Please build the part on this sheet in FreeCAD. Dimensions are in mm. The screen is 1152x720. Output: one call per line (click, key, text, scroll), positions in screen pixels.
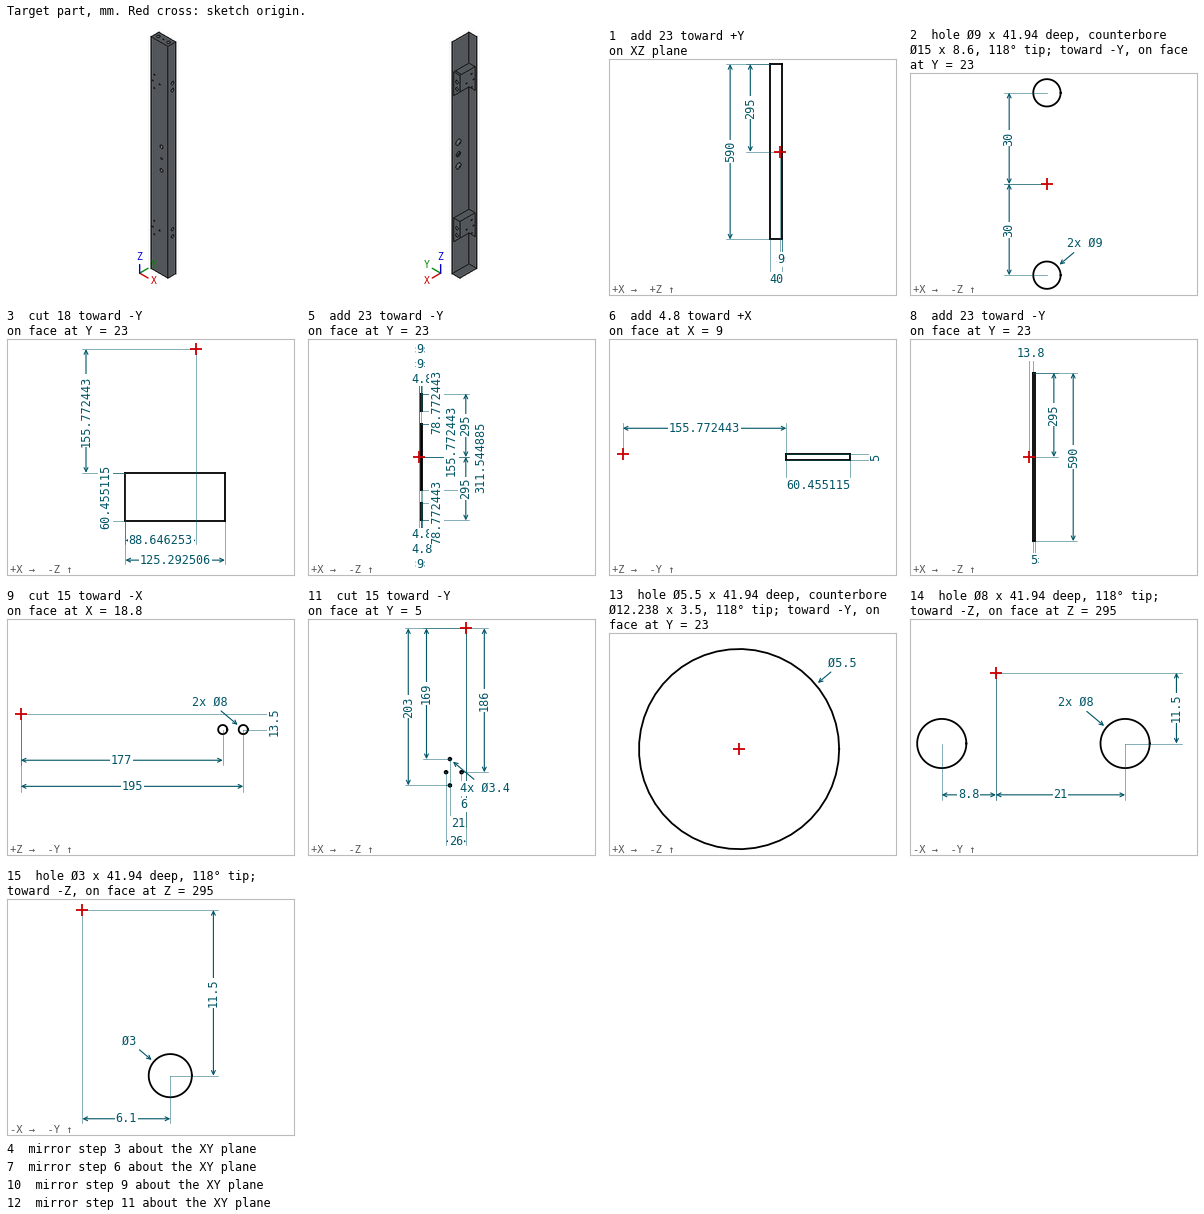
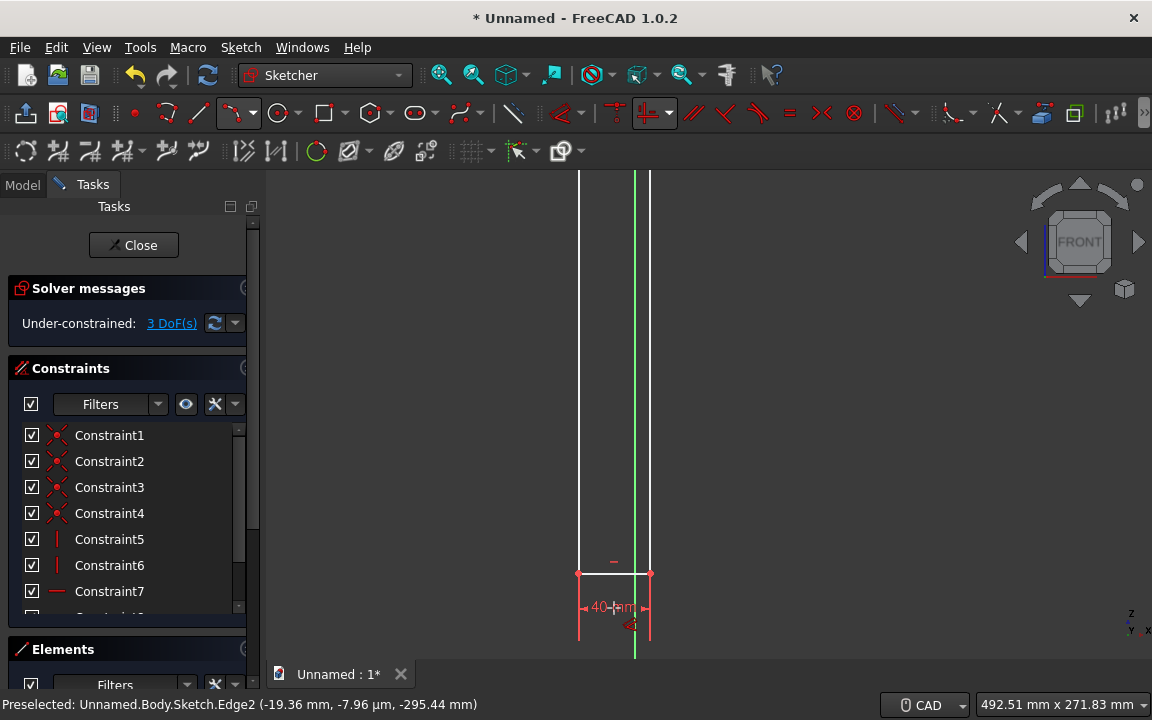
scroll(650, 574, up, 5)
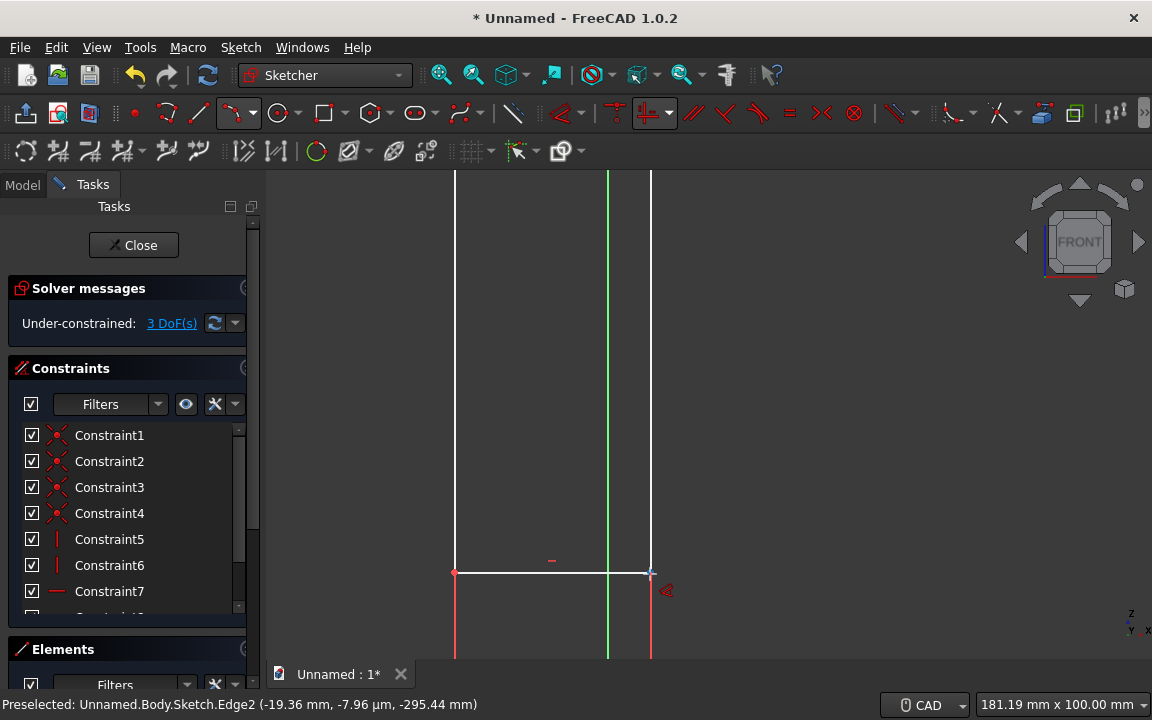
click(651, 573)
click(629, 607)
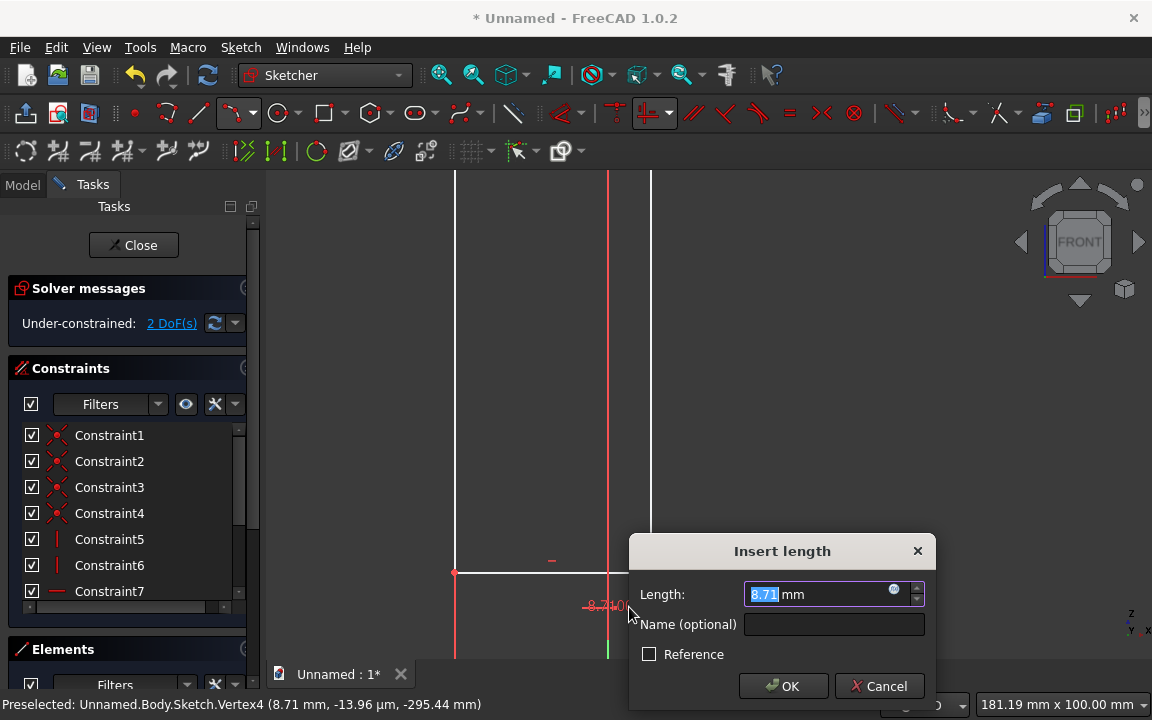
text(9)
key(Return)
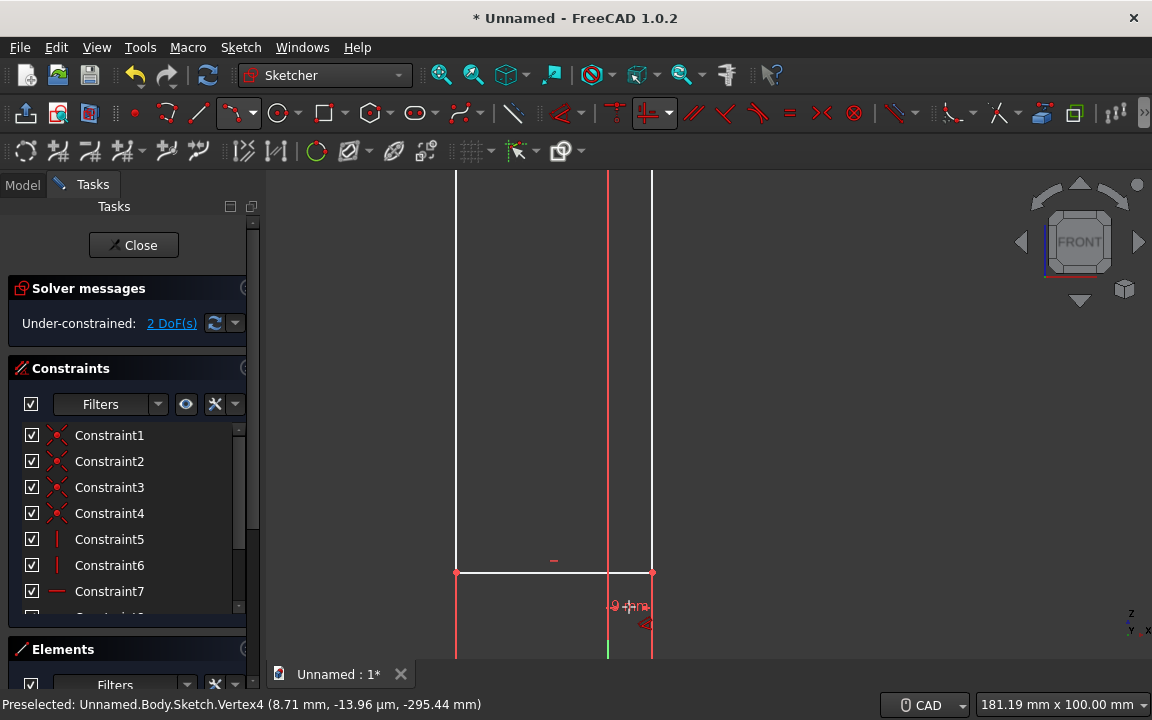
scroll(651, 575, down, 11)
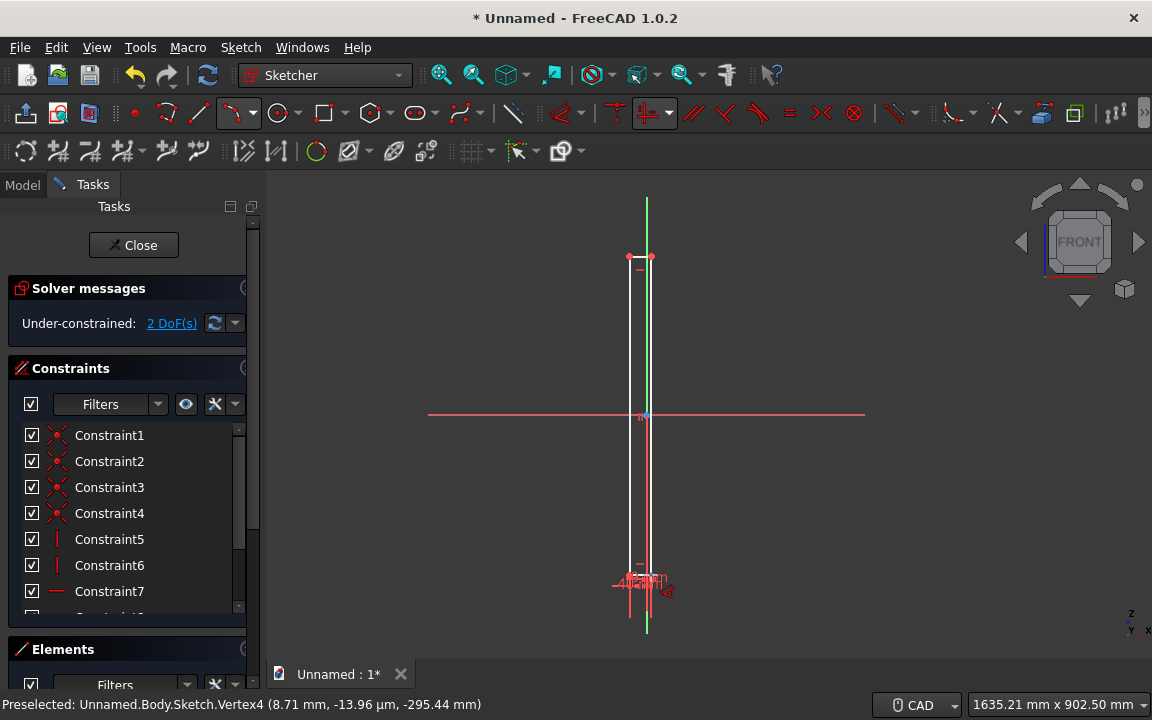
click(630, 352)
click(596, 343)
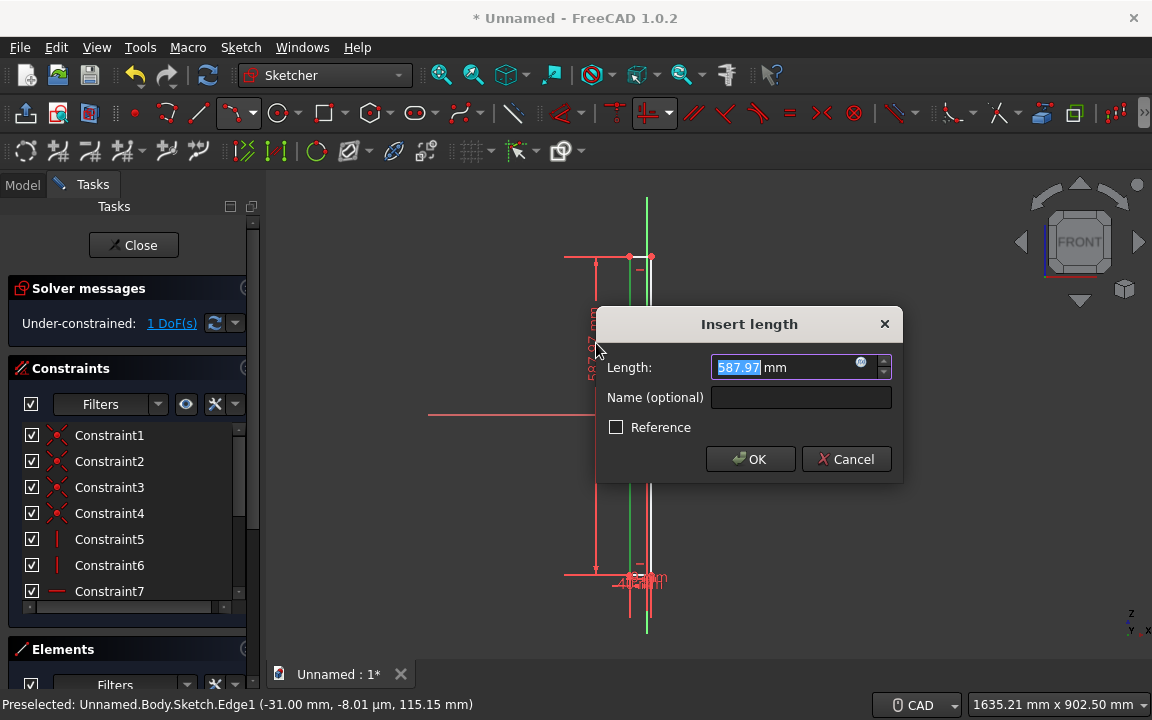
text(590)
key(Return)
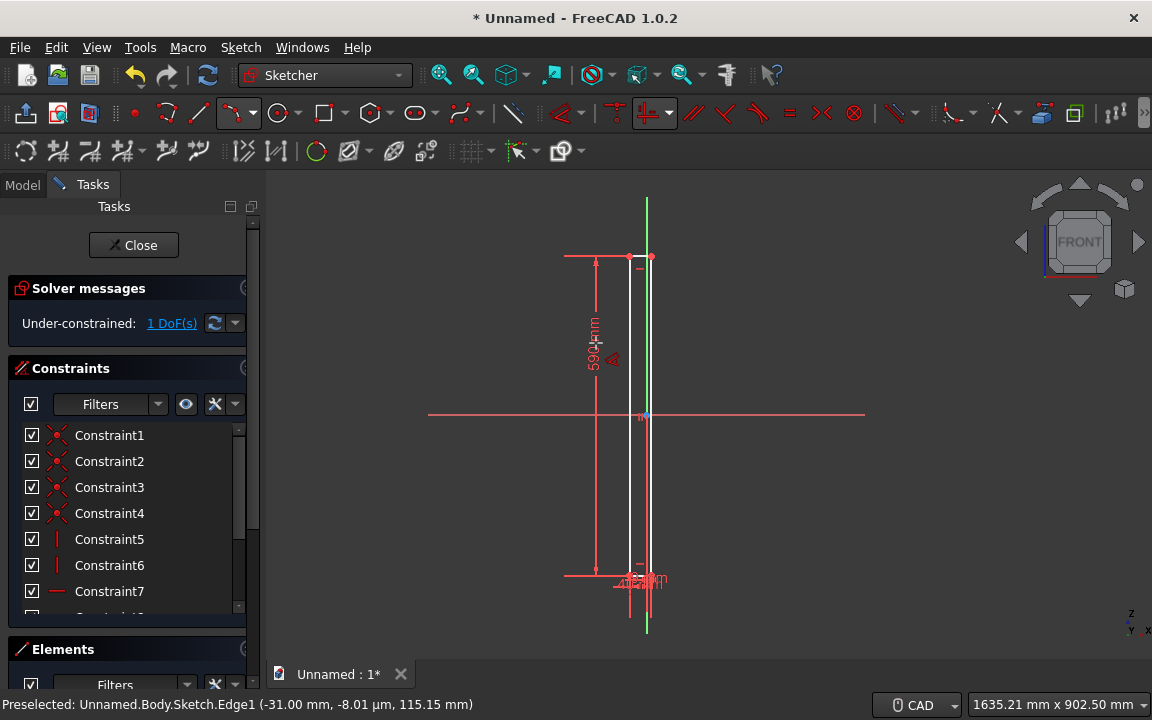
click(630, 256)
click(596, 299)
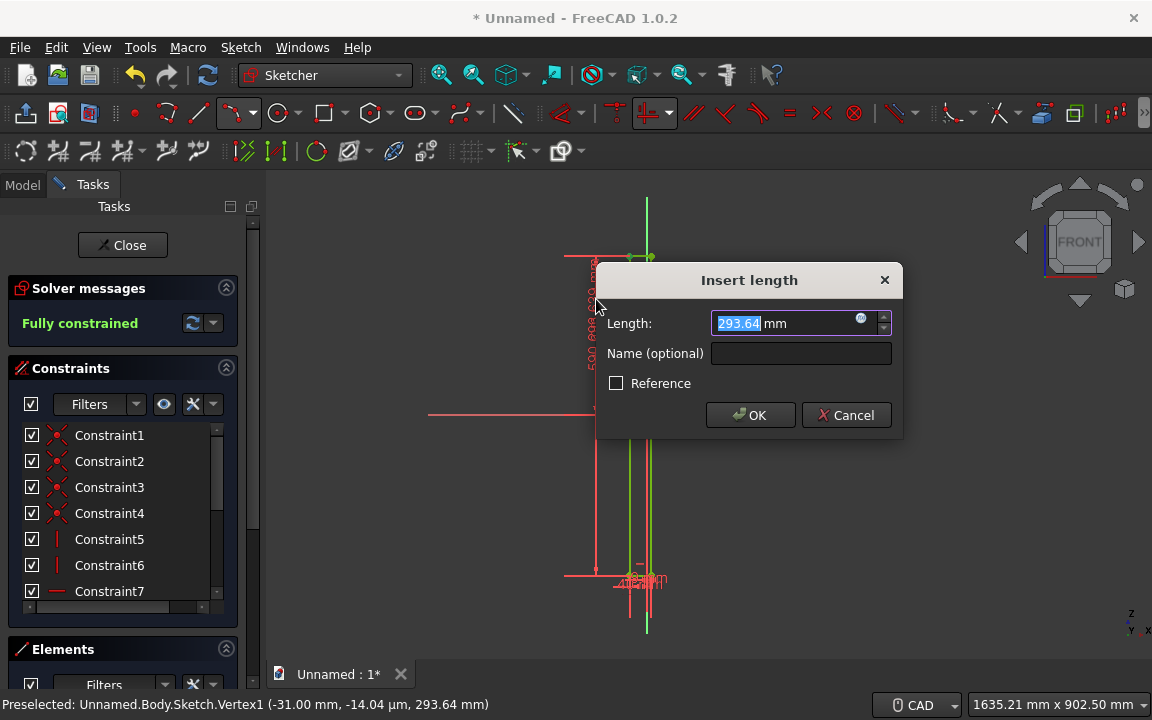
text(295)
key(Return)
key(Escape)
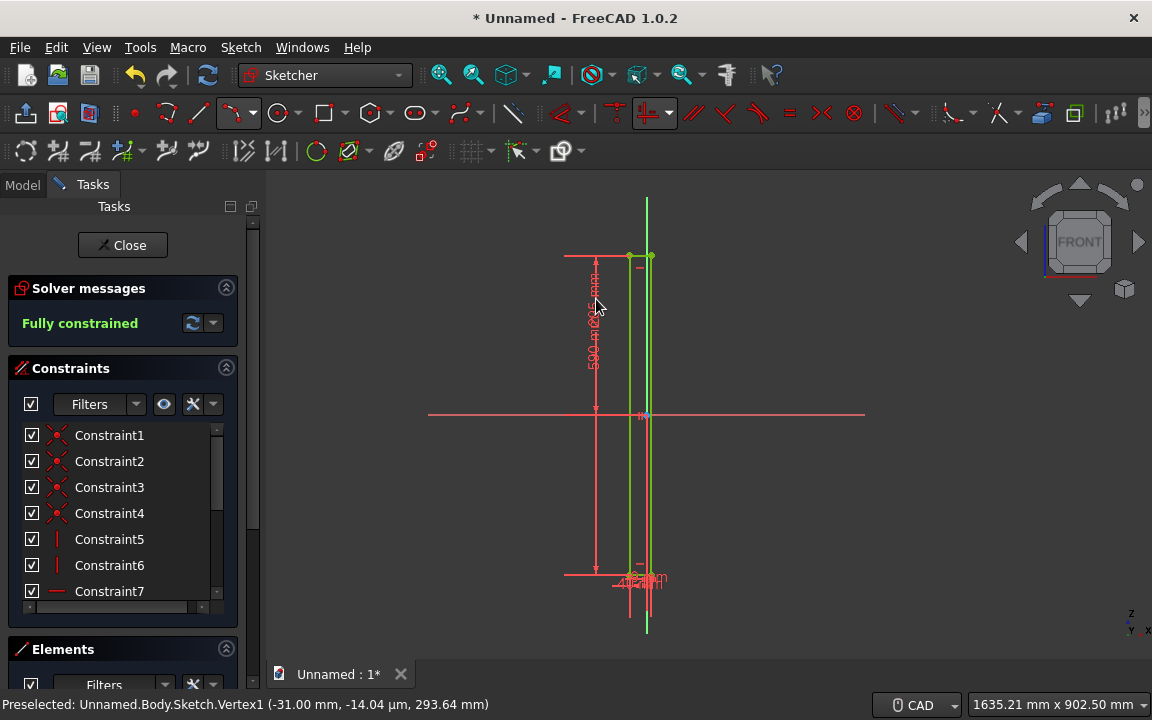
click(123, 245)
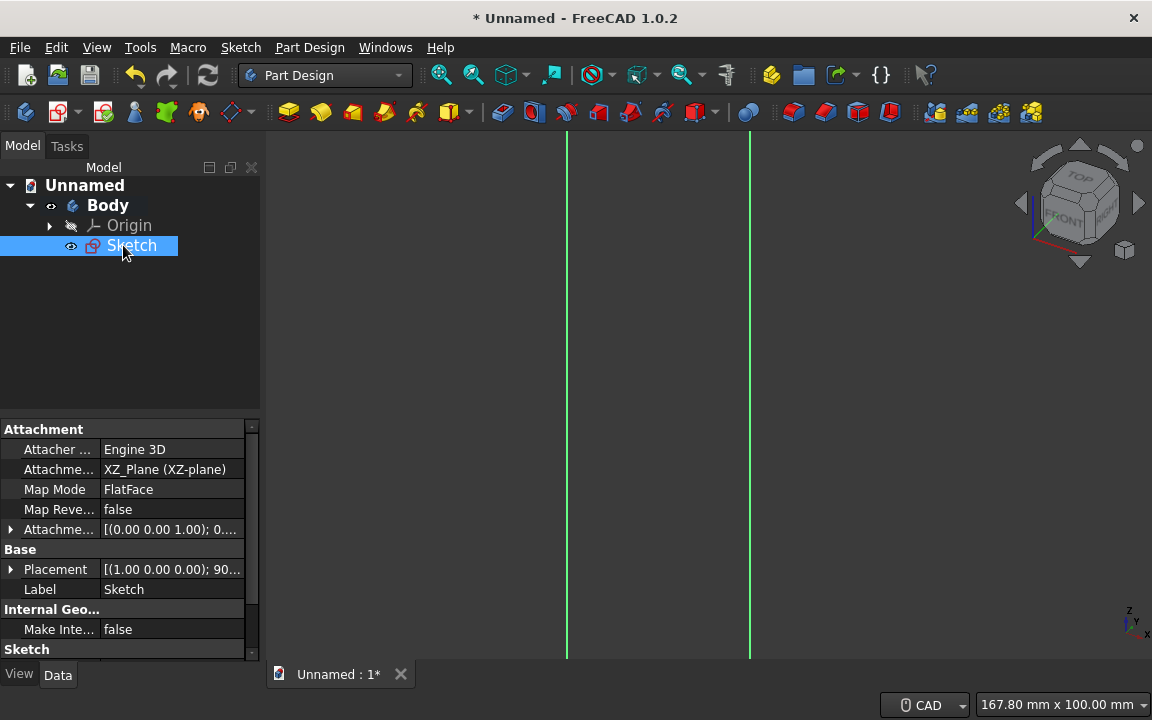
click(290, 112)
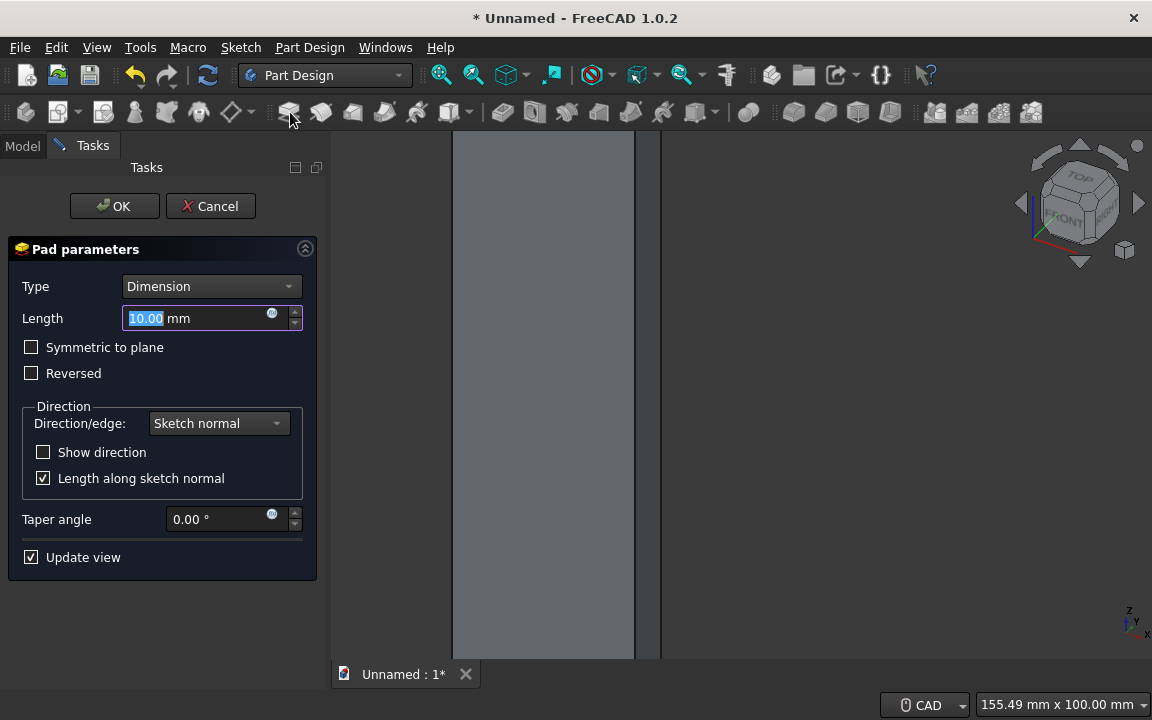
text(23)
key(Tab)